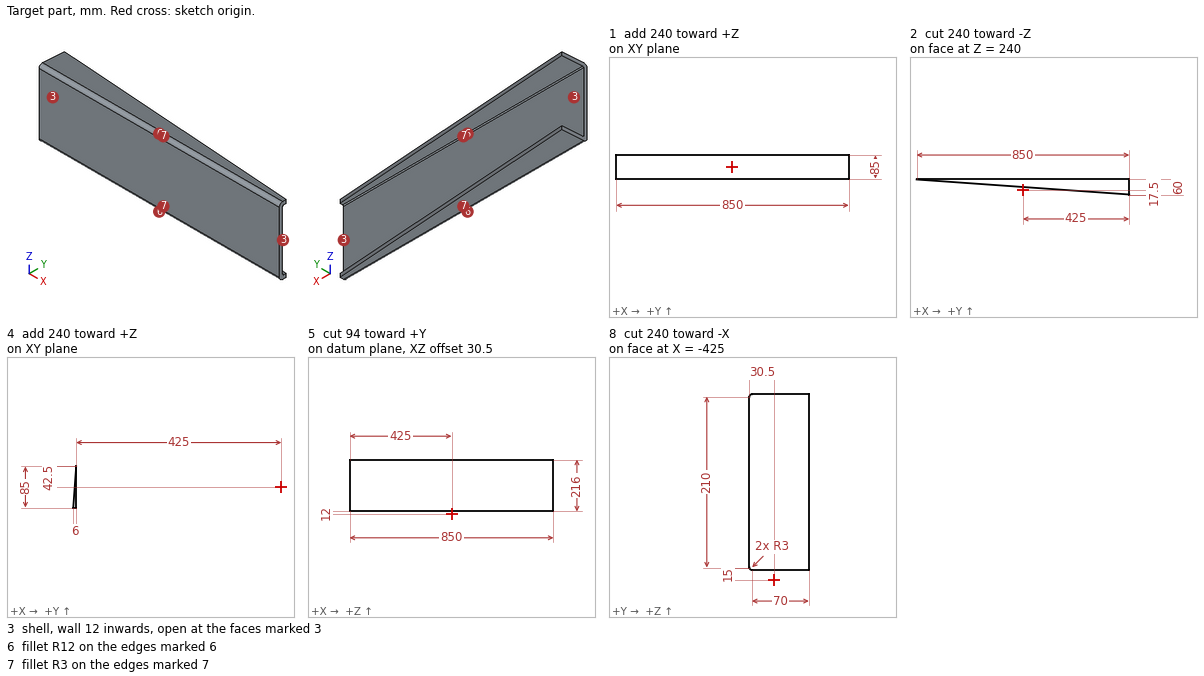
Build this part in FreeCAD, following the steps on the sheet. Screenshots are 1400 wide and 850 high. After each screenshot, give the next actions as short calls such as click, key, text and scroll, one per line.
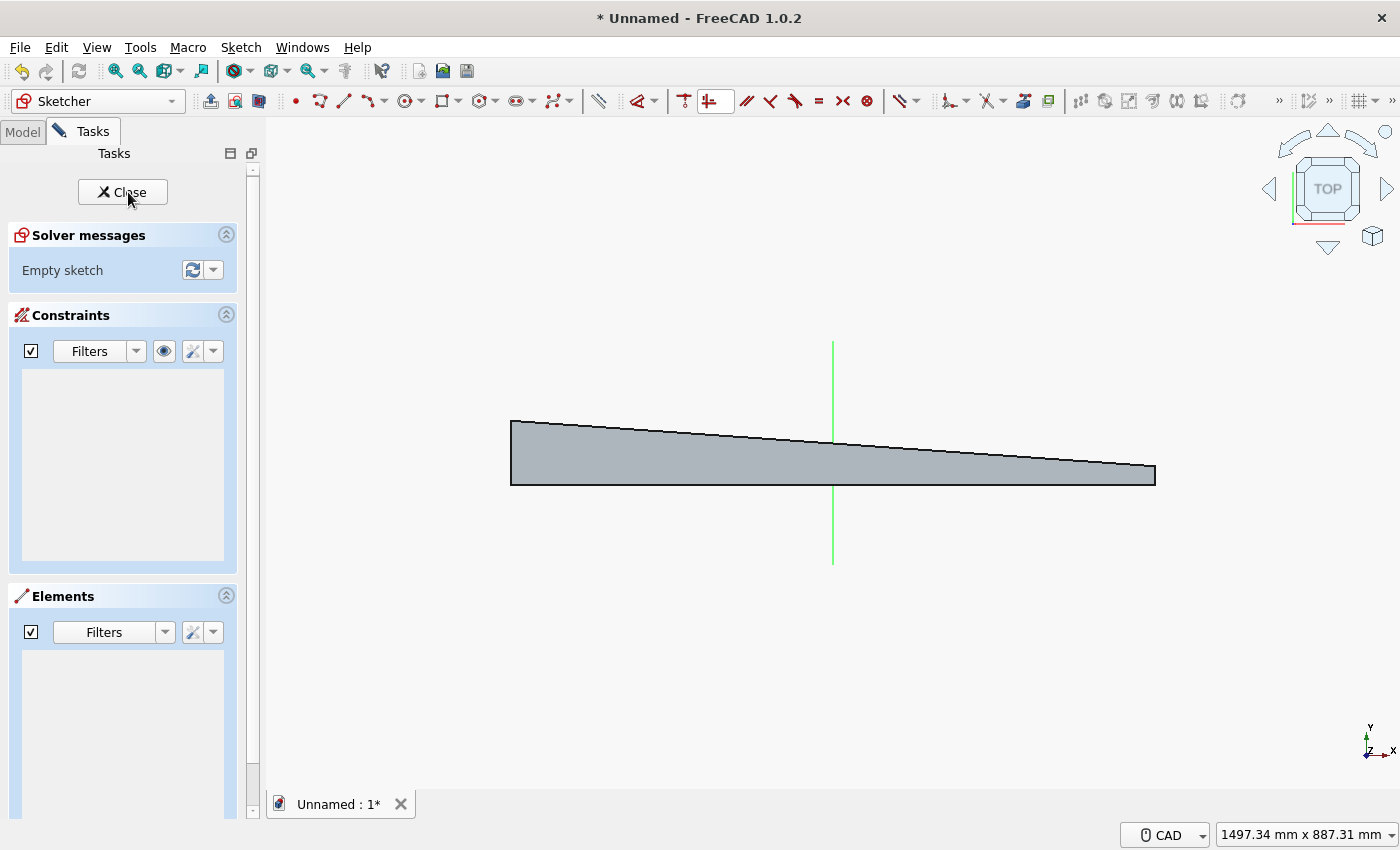
key(q)
key(s)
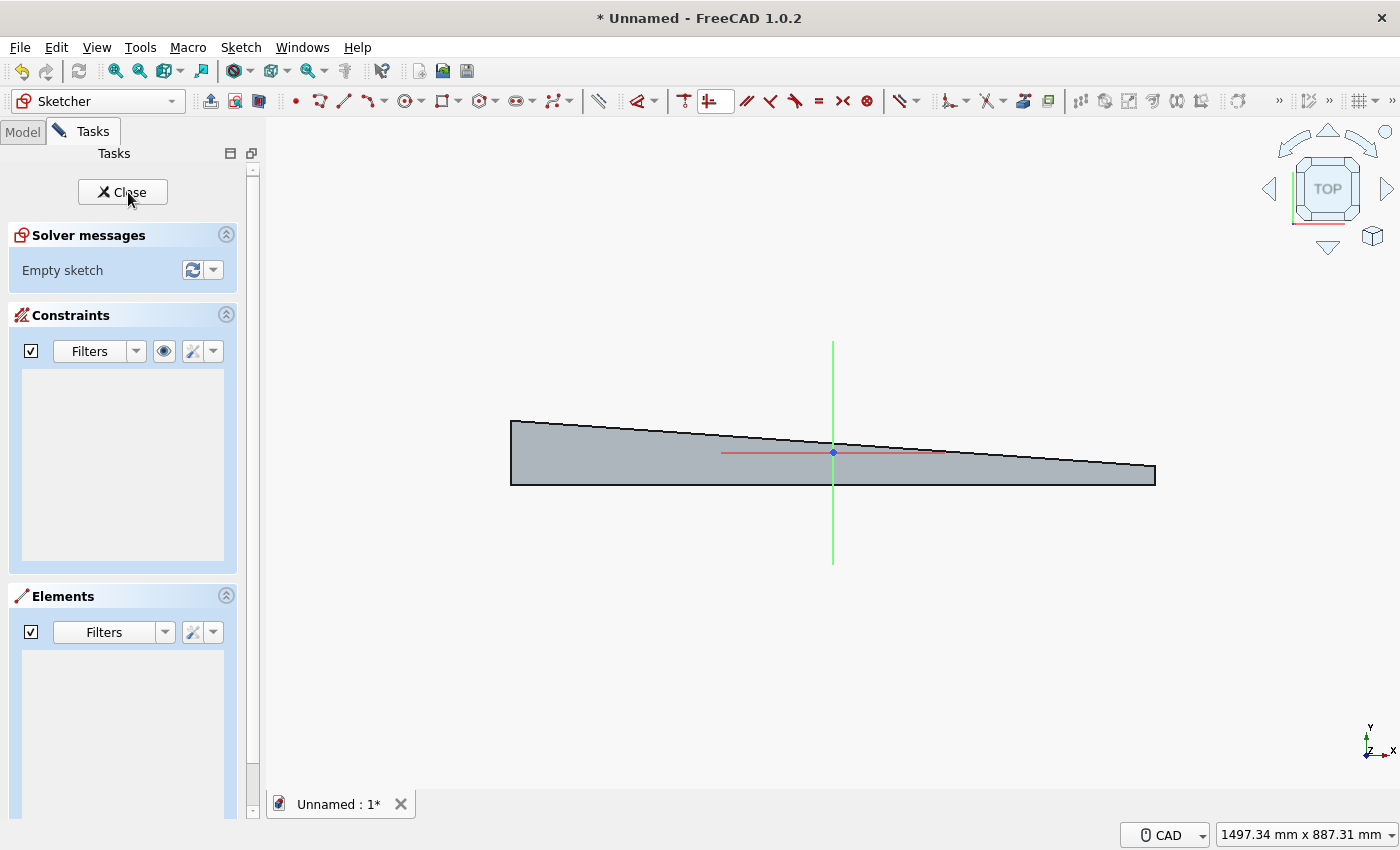
scroll(469, 453, up, 10)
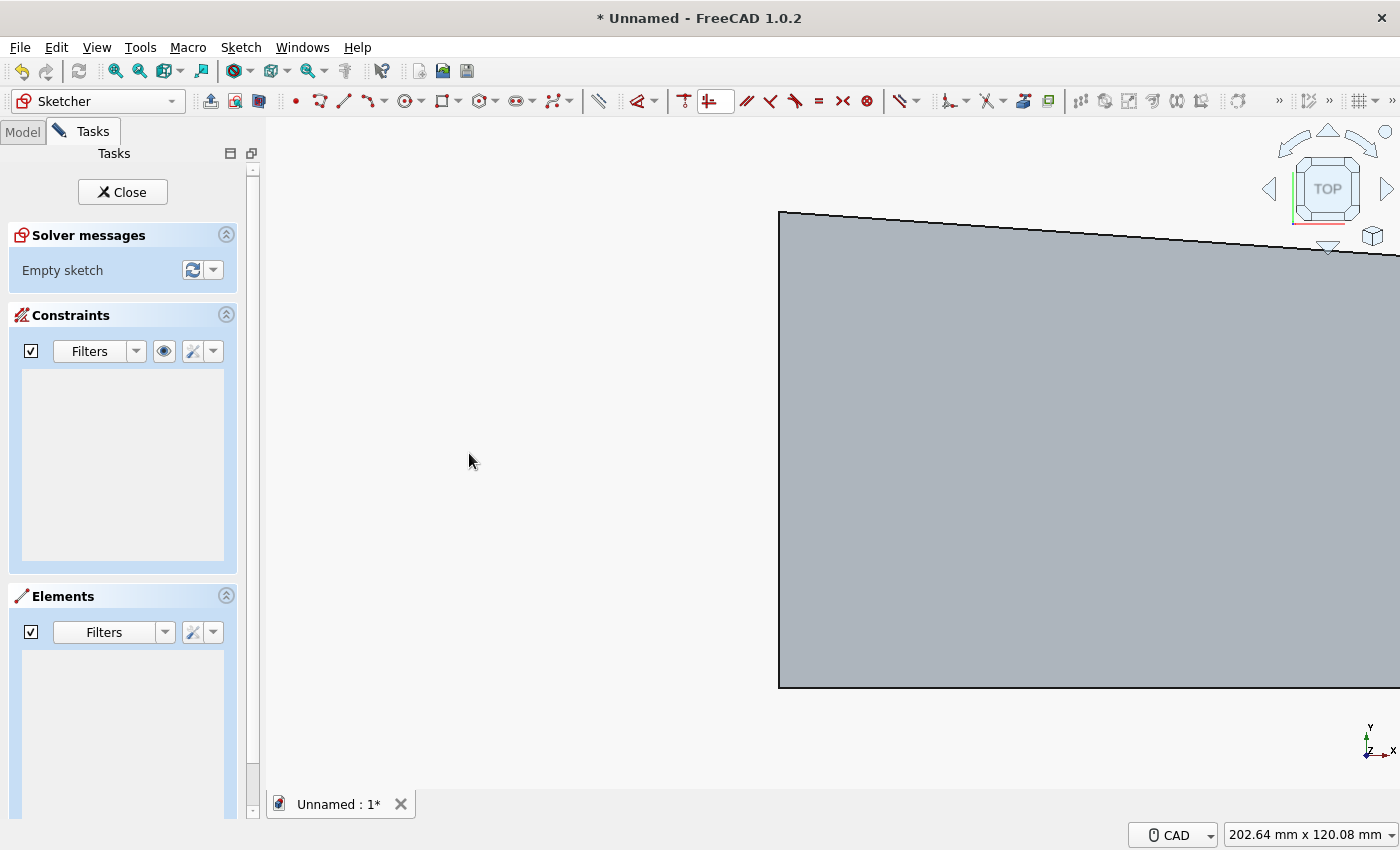
key(g)
key(m)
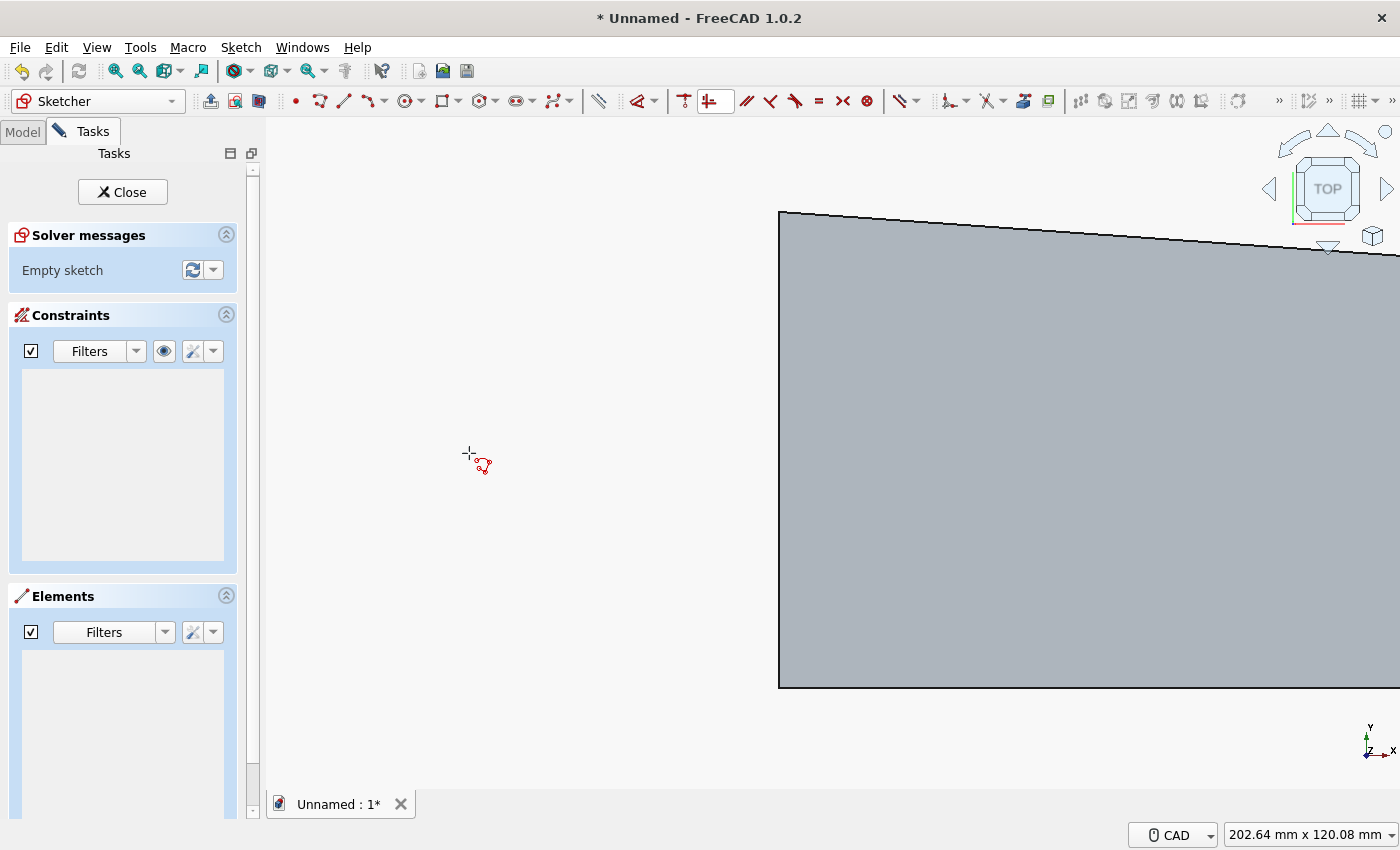
click(779, 212)
click(779, 688)
click(746, 688)
click(779, 213)
key(Escape)
key(Escape)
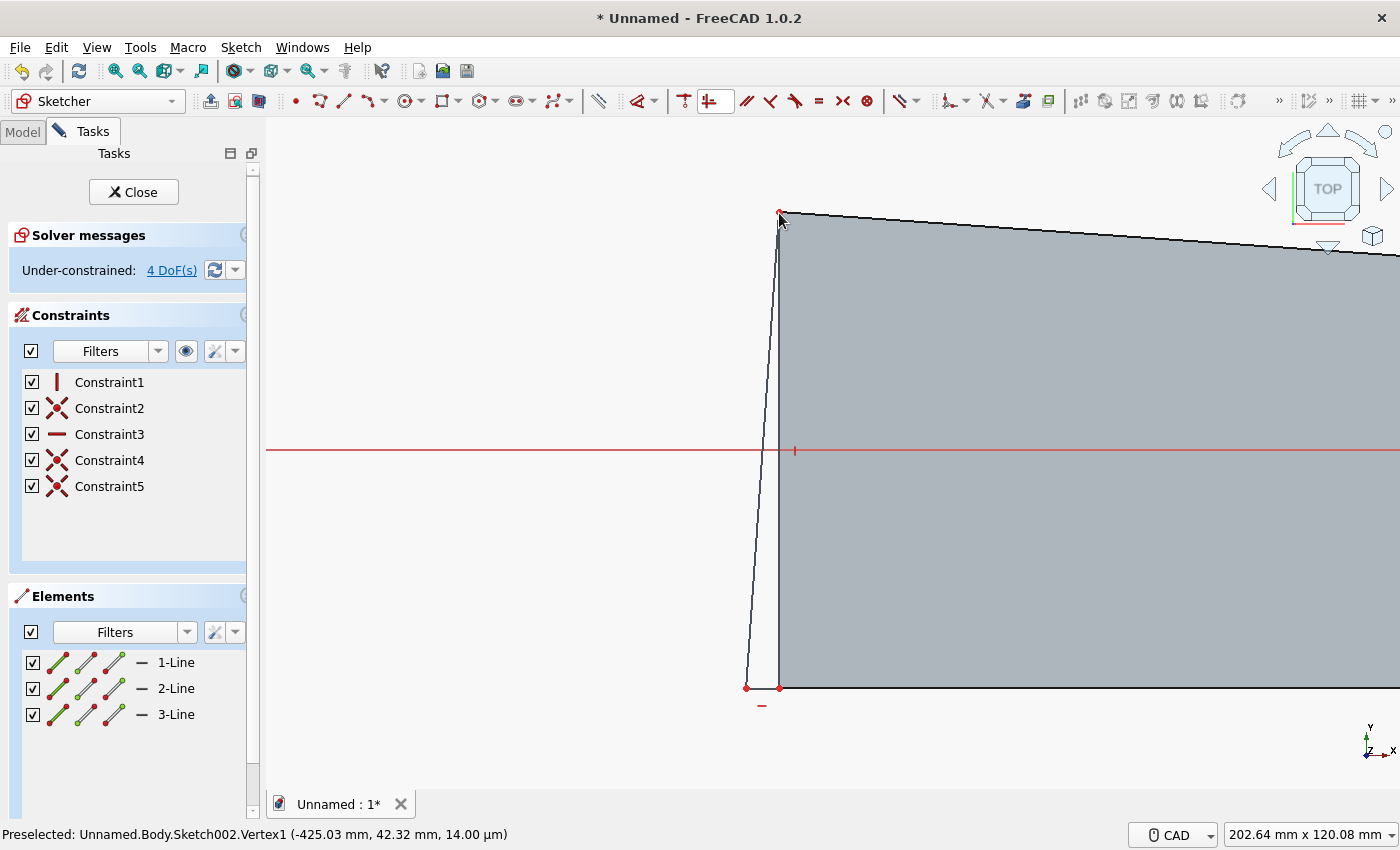
key(d)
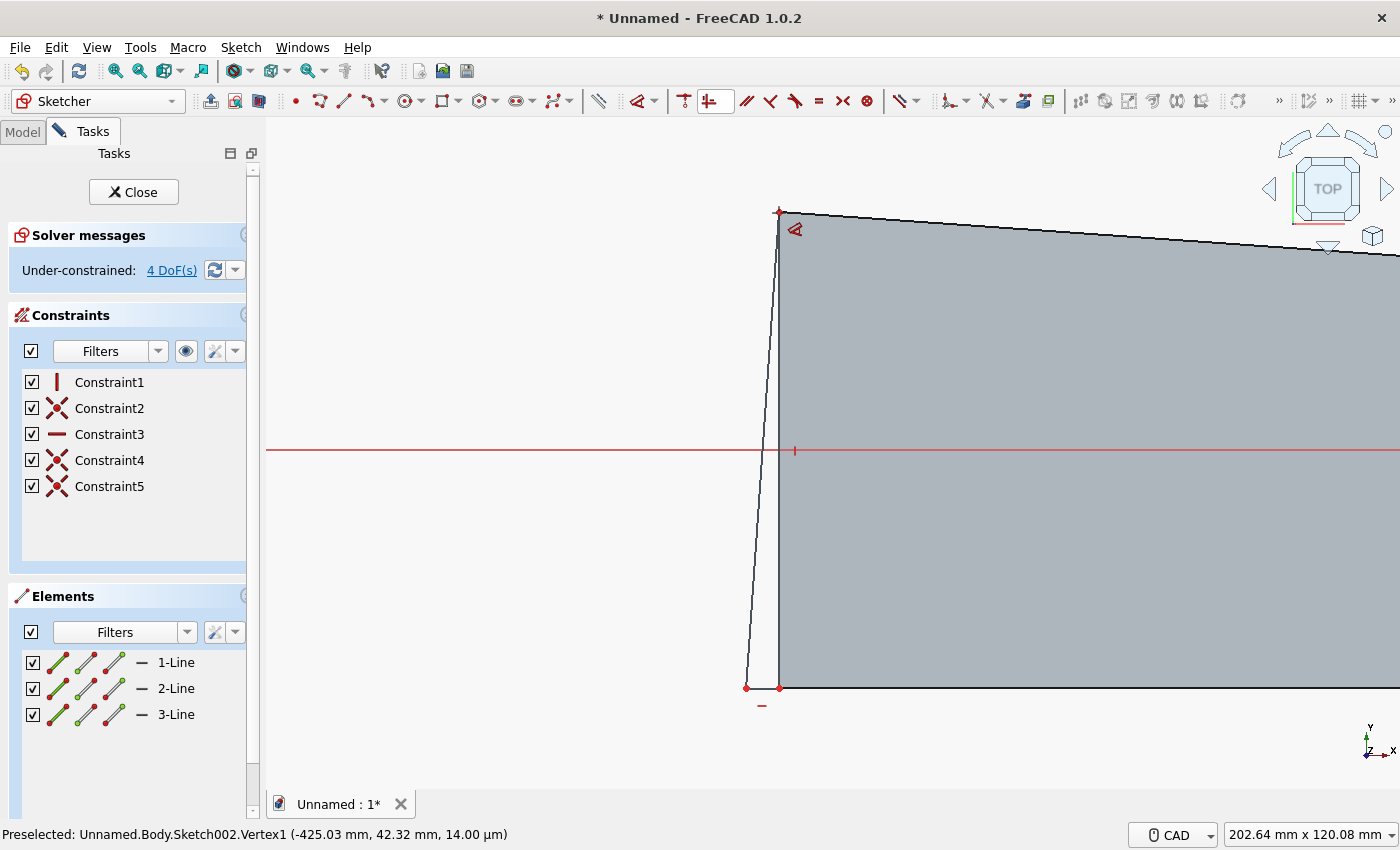
scroll(769, 689, up, 2)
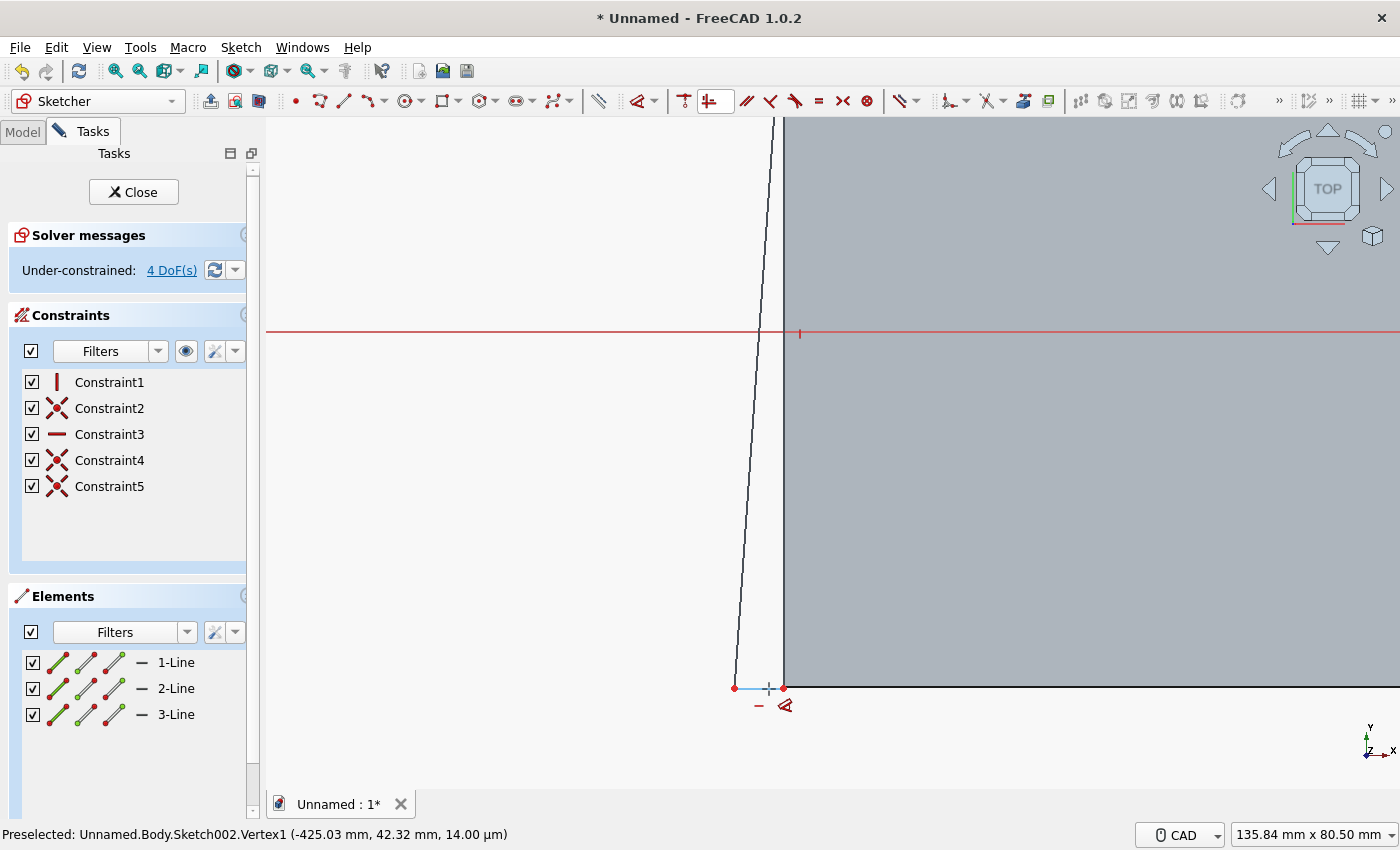
click(769, 689)
click(759, 723)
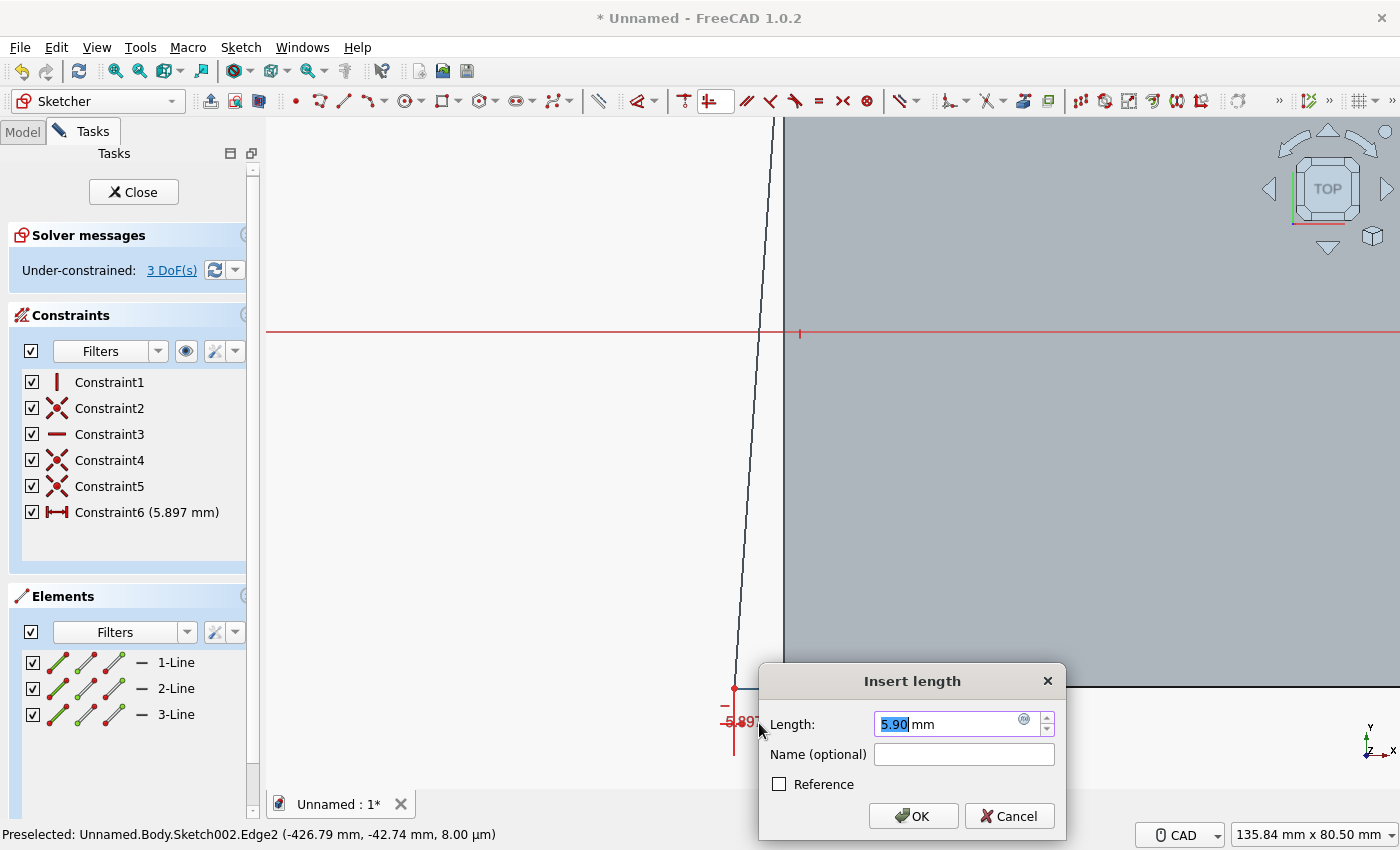
text(6)
key(Return)